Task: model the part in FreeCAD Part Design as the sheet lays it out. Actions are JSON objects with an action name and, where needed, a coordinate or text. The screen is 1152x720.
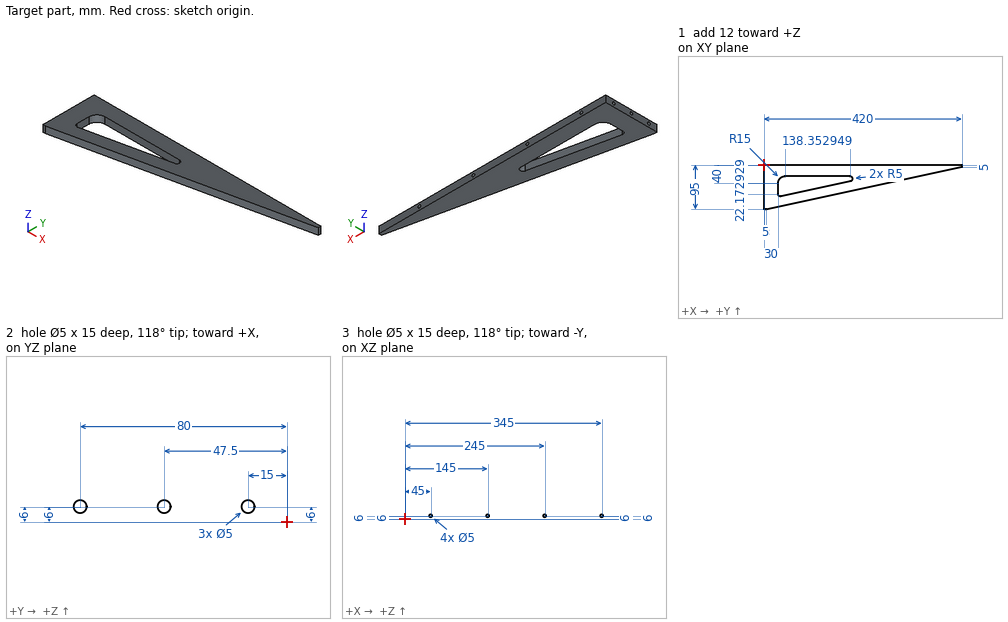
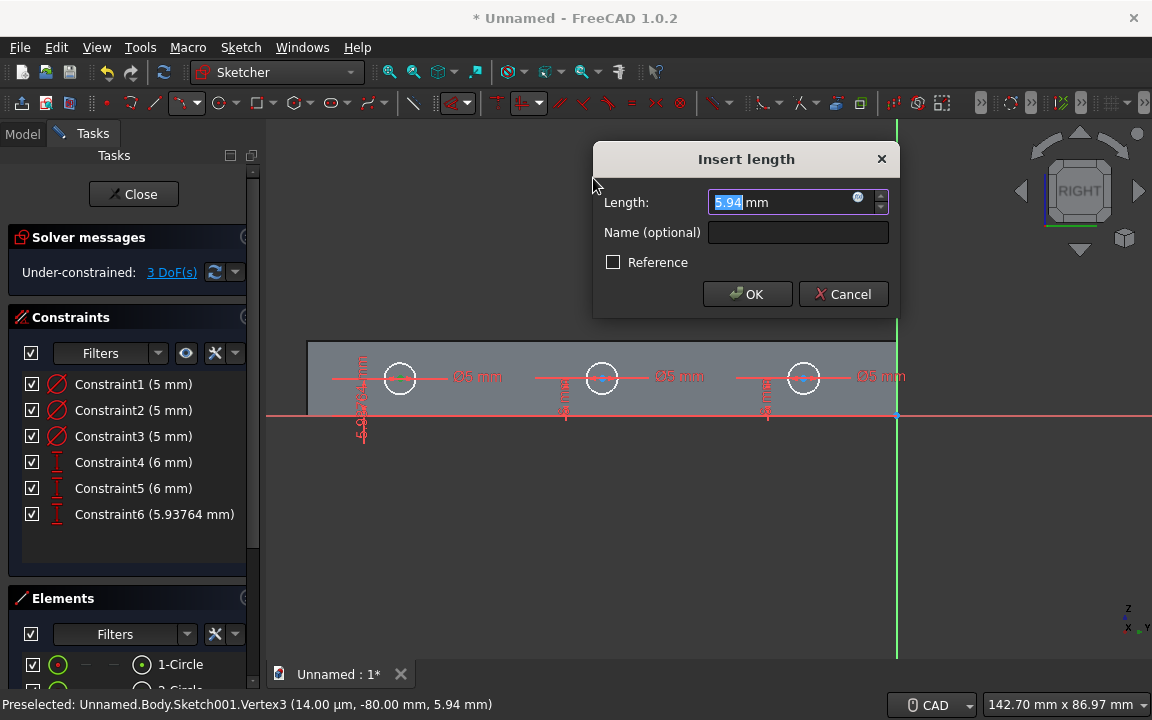
{"action": "type", "text": "6"}
{"action": "key", "text": "Return"}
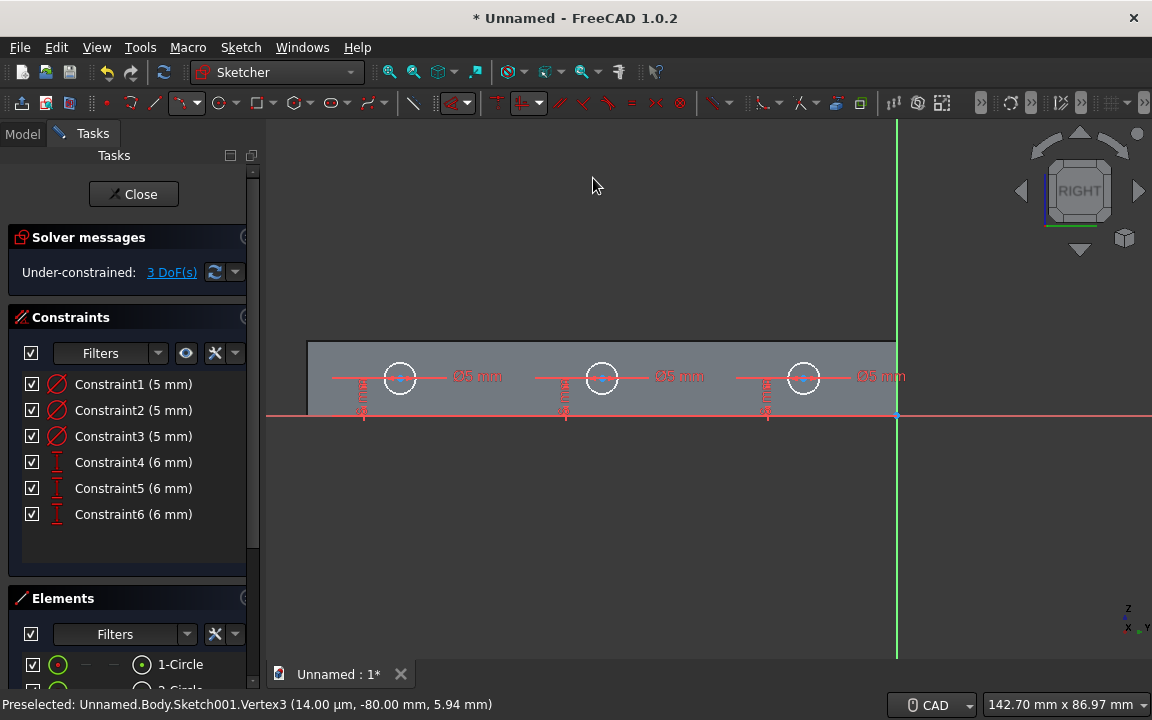
{"action": "left_click", "coordinate": [804, 378]}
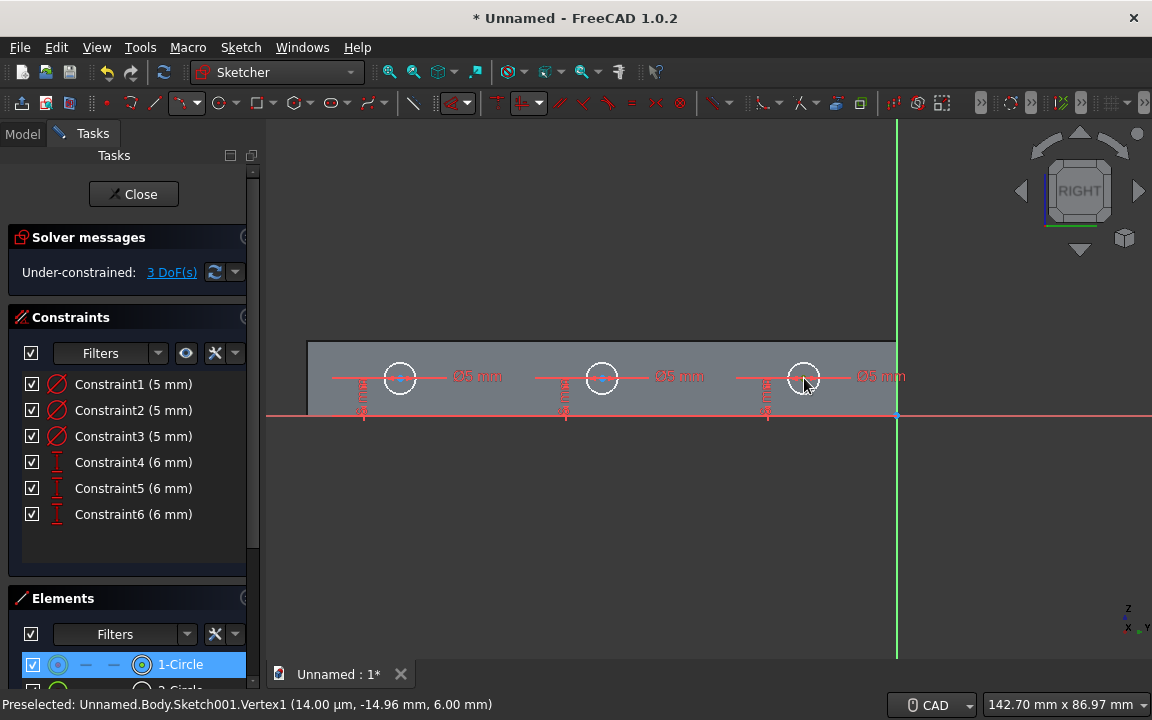
{"action": "left_click", "coordinate": [470, 104]}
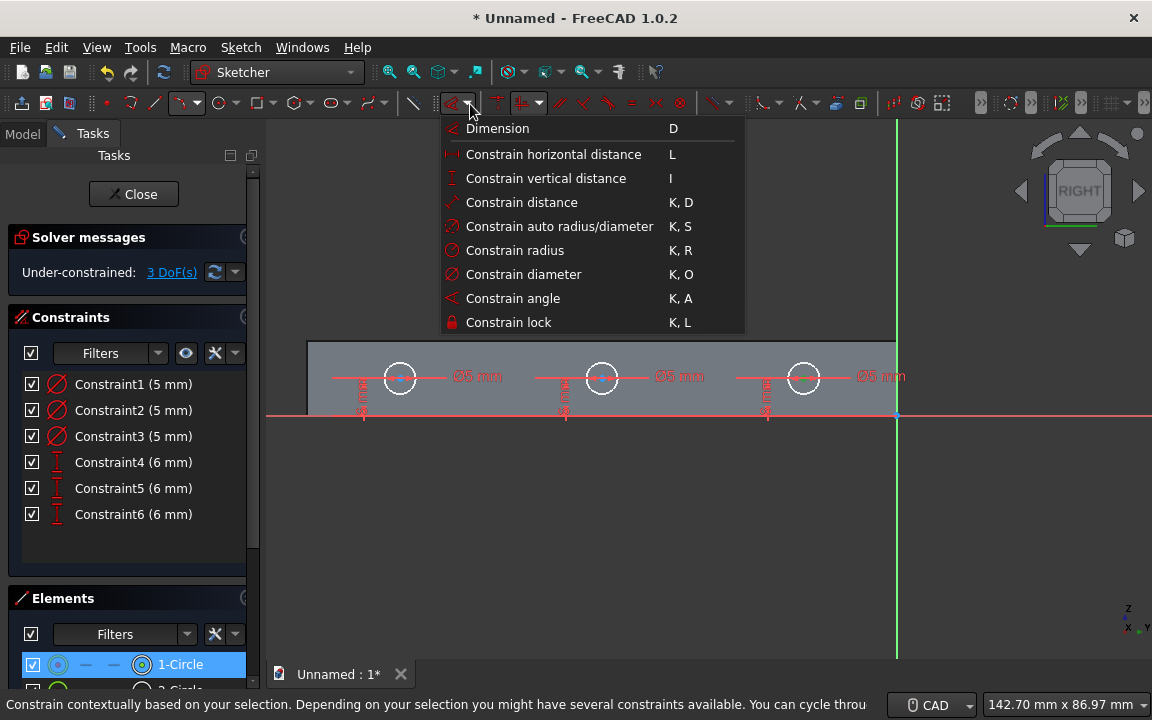
{"action": "left_click", "coordinate": [593, 154]}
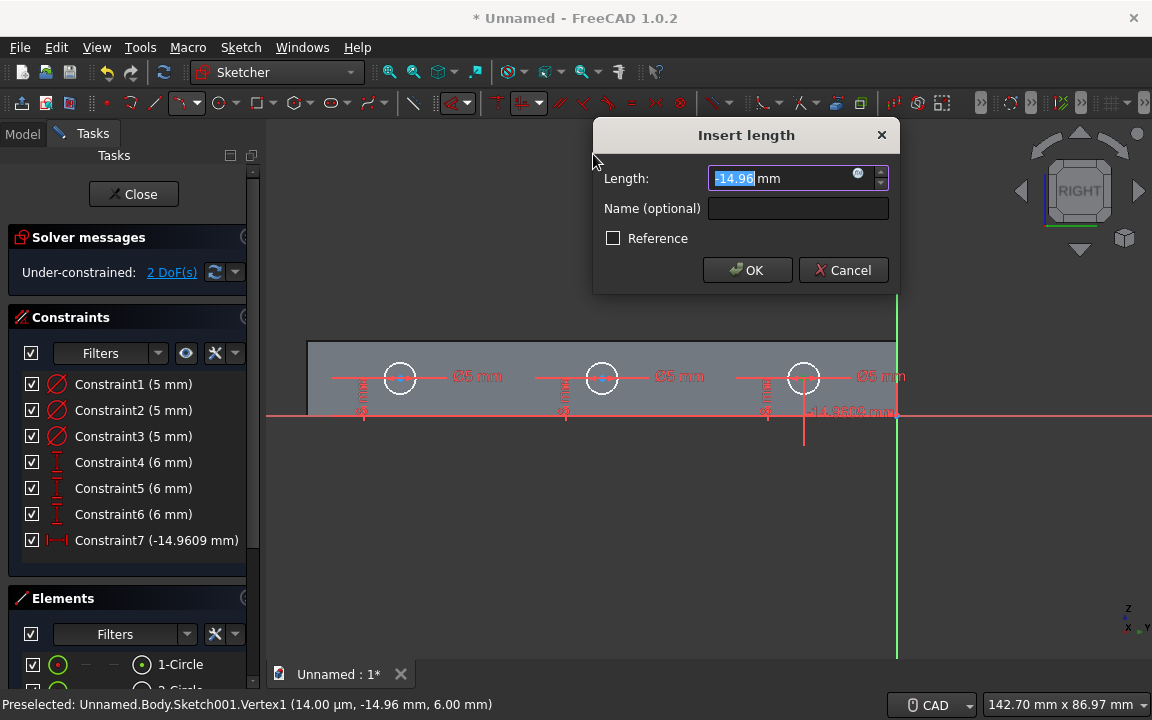
{"action": "type", "text": "-15"}
{"action": "key", "text": "Return"}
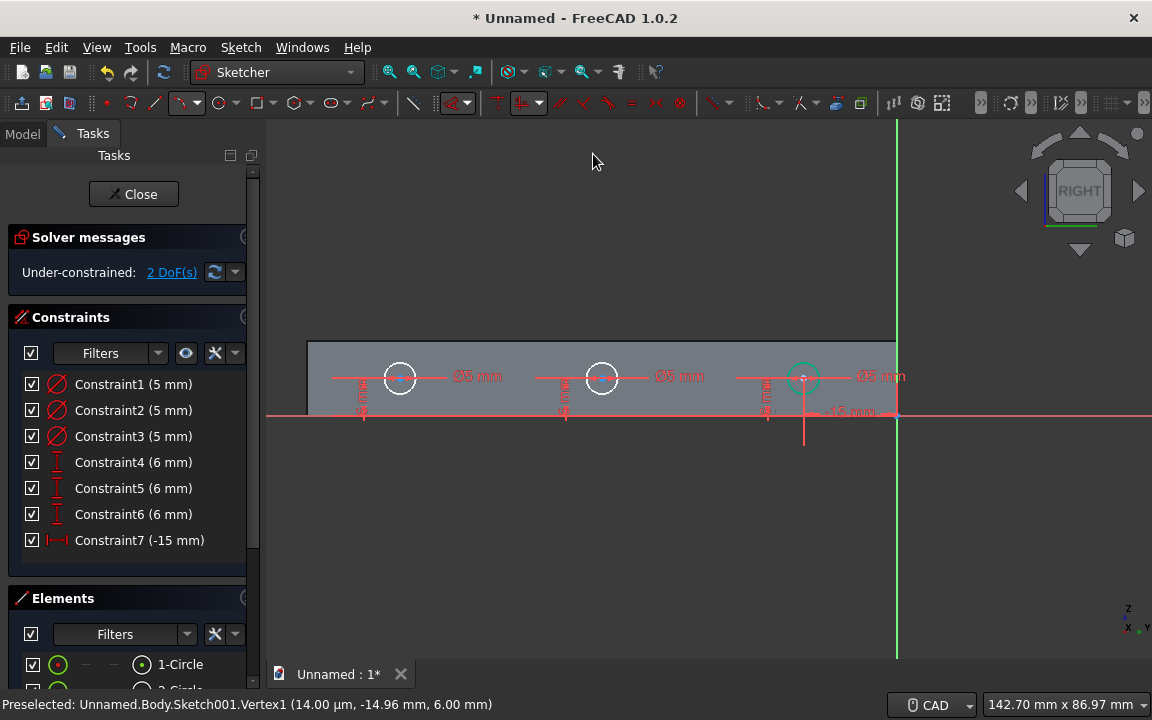
{"action": "left_click", "coordinate": [400, 378]}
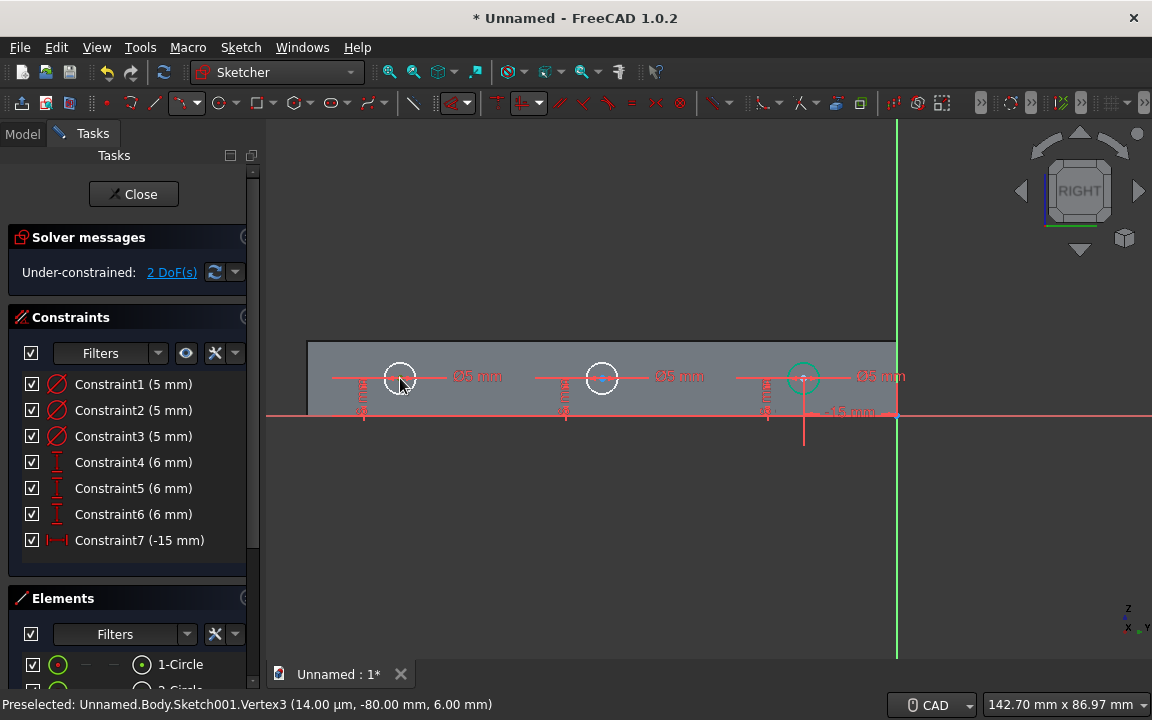
{"action": "key", "text": "l"}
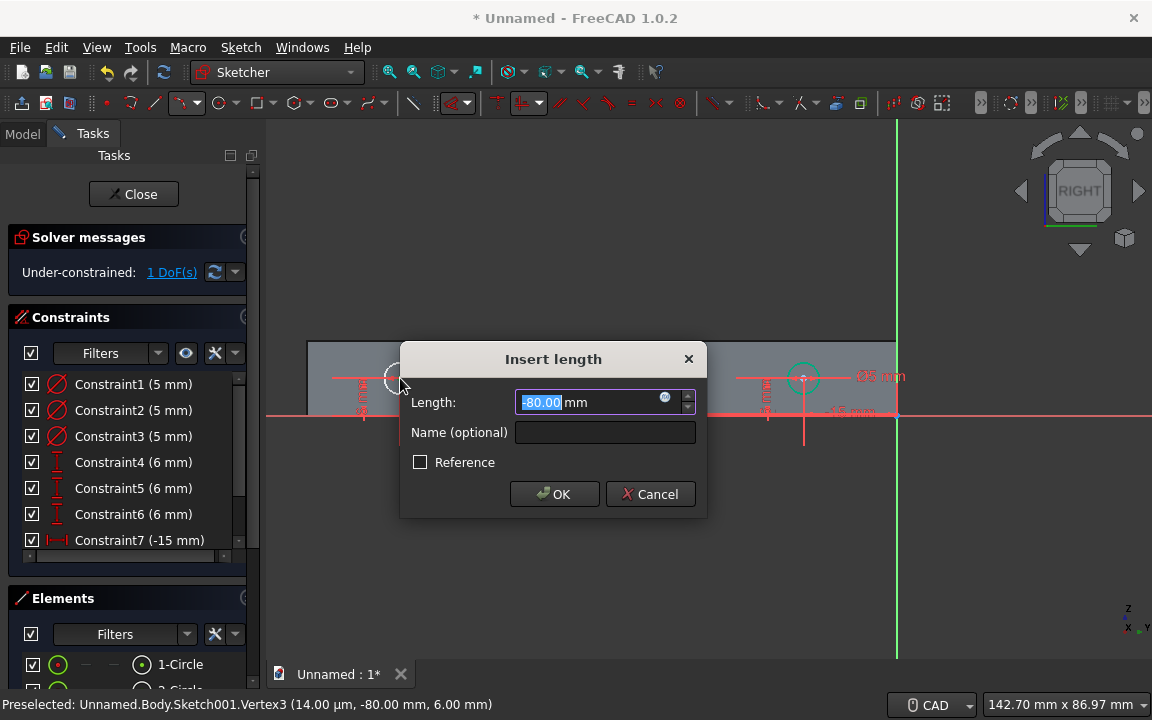
{"action": "type", "text": "-80"}
{"action": "key", "text": "Return"}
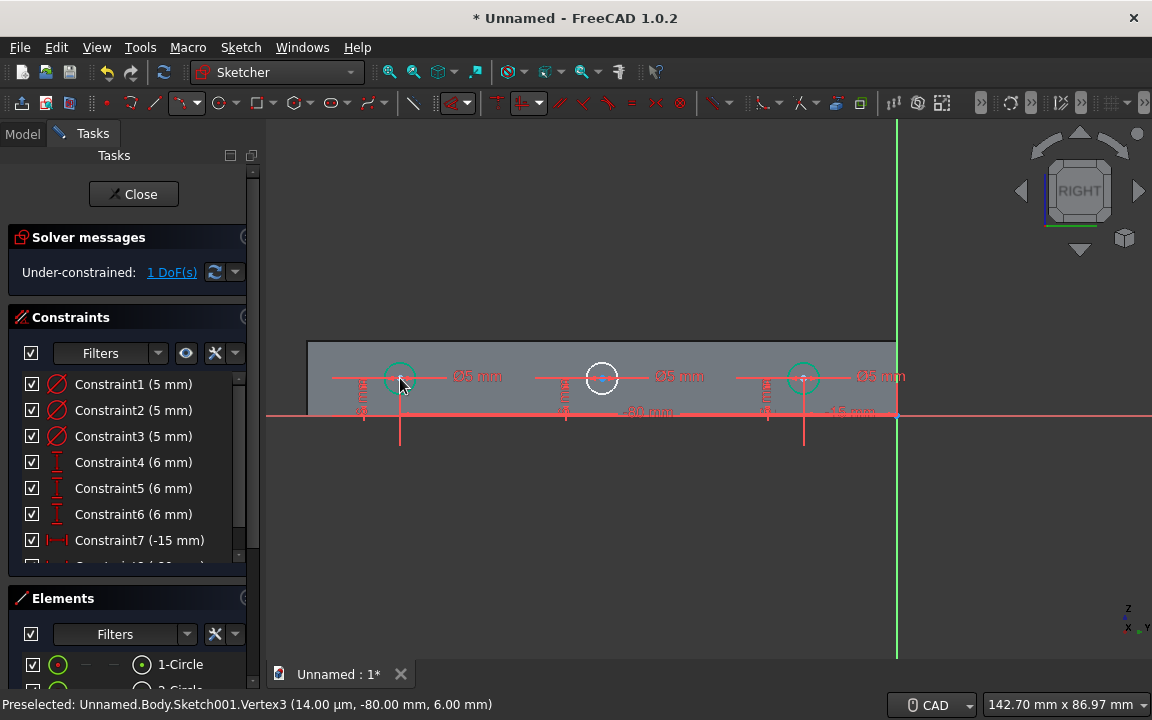
{"action": "left_click", "coordinate": [602, 378]}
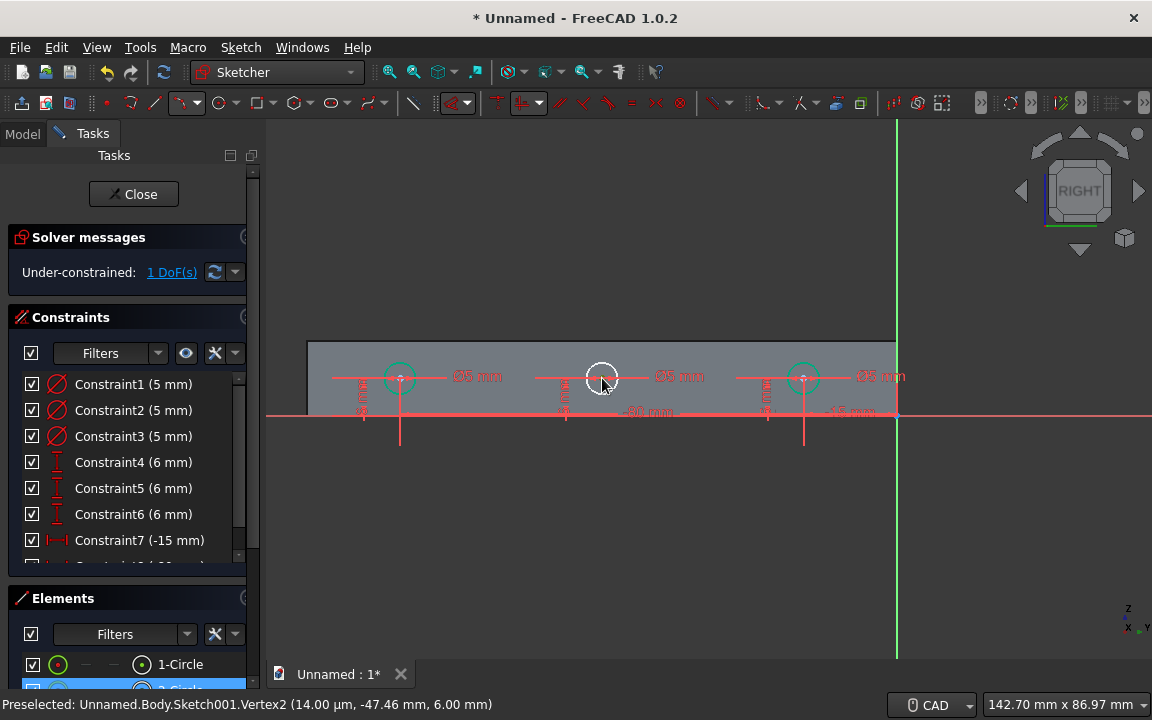
{"action": "left_click", "coordinate": [470, 104]}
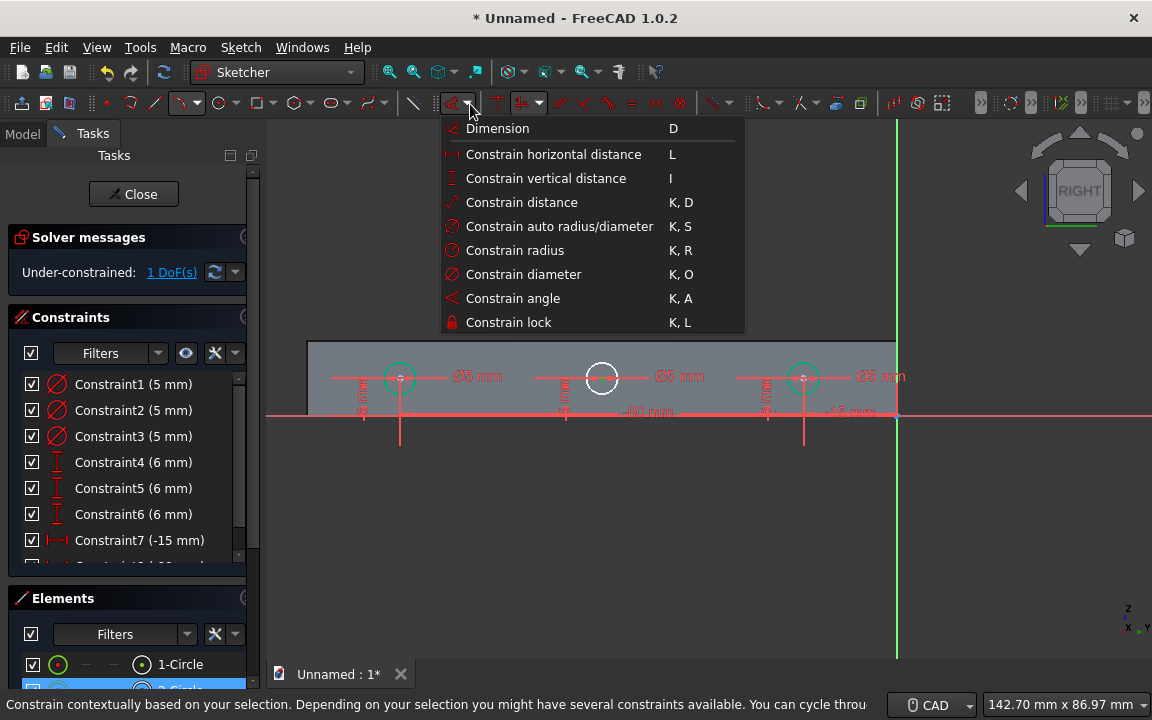
{"action": "left_click", "coordinate": [593, 154]}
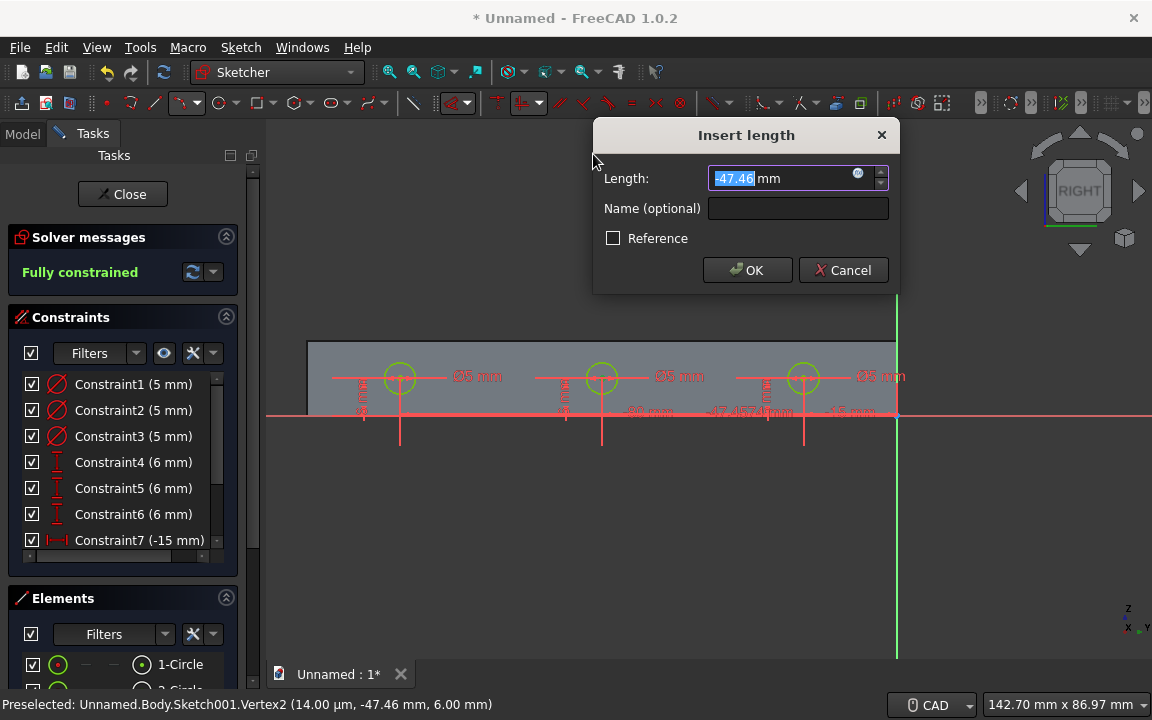
{"action": "type", "text": "-47.5"}
{"action": "key", "text": "Return"}